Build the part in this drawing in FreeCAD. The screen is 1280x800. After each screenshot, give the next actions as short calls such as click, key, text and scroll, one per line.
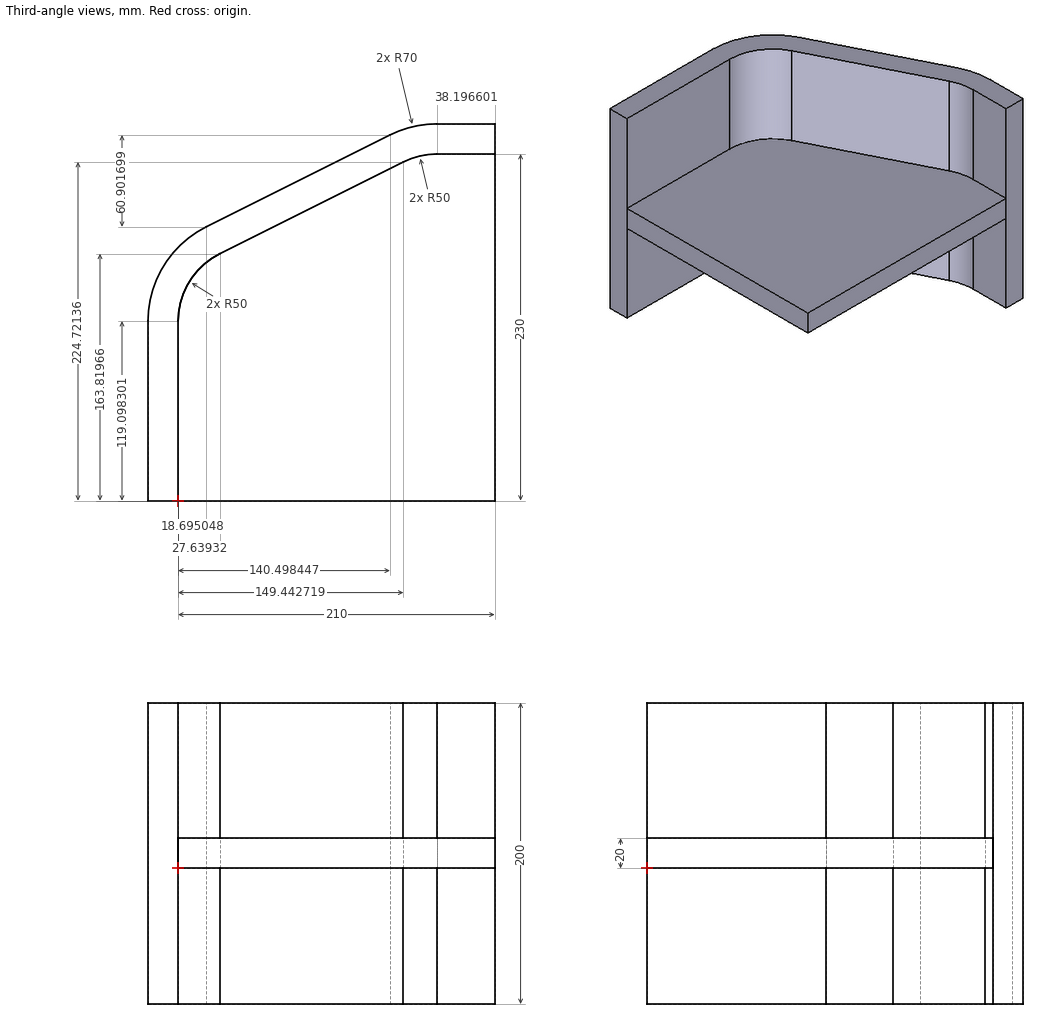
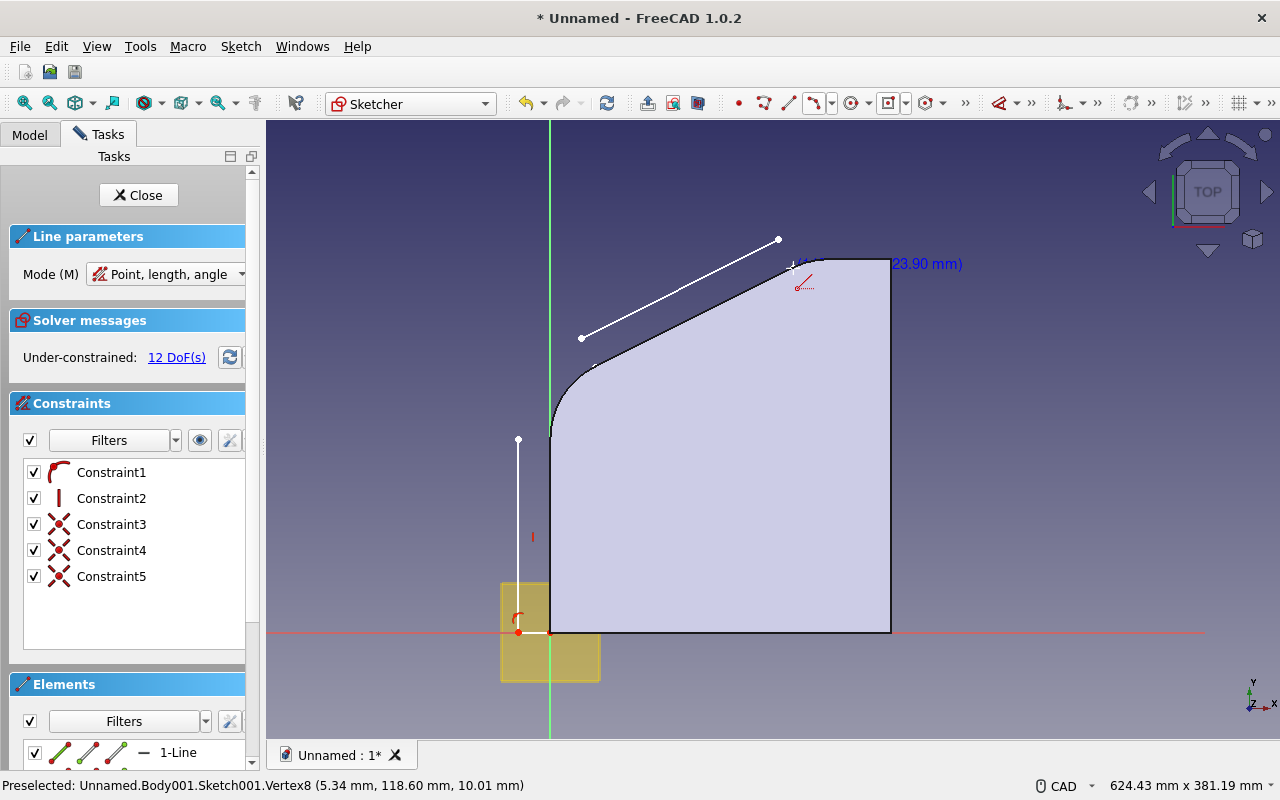
click(764, 104)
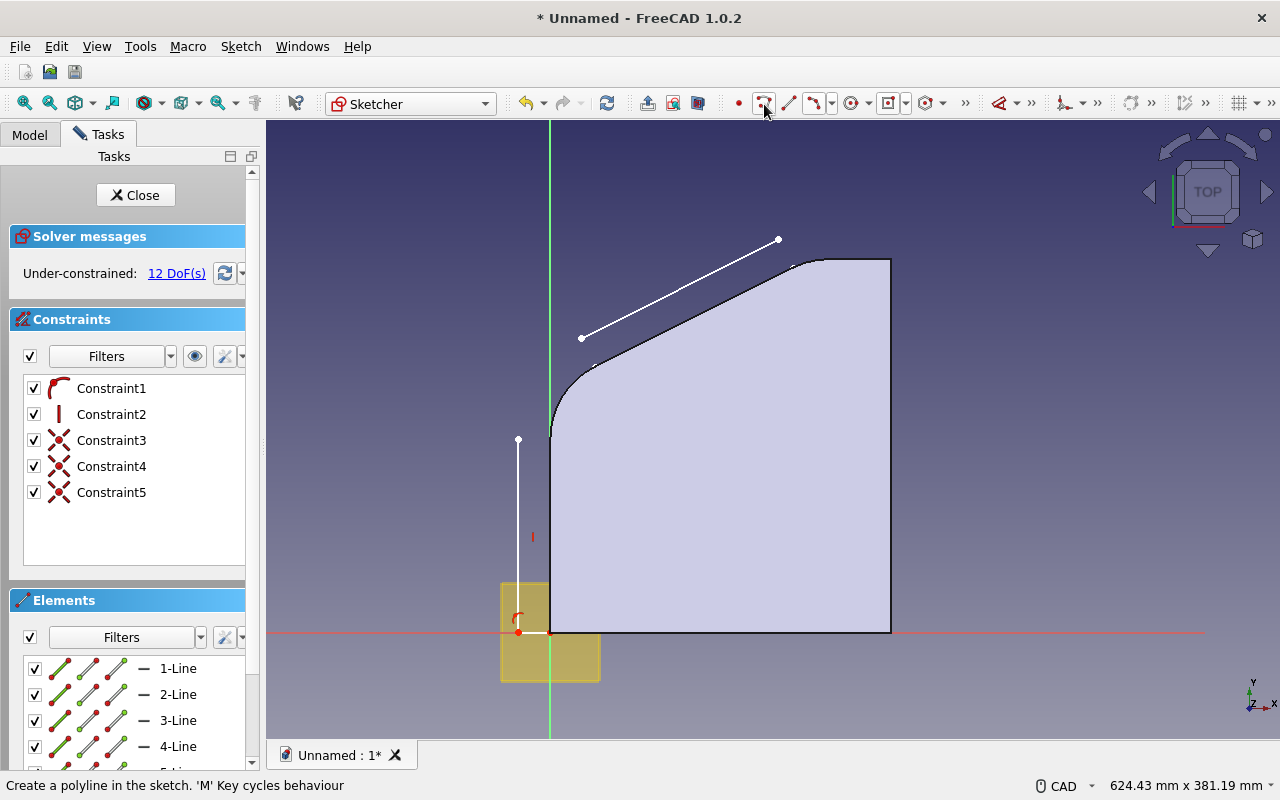
click(829, 259)
click(891, 259)
click(891, 227)
click(829, 227)
right_click(829, 227)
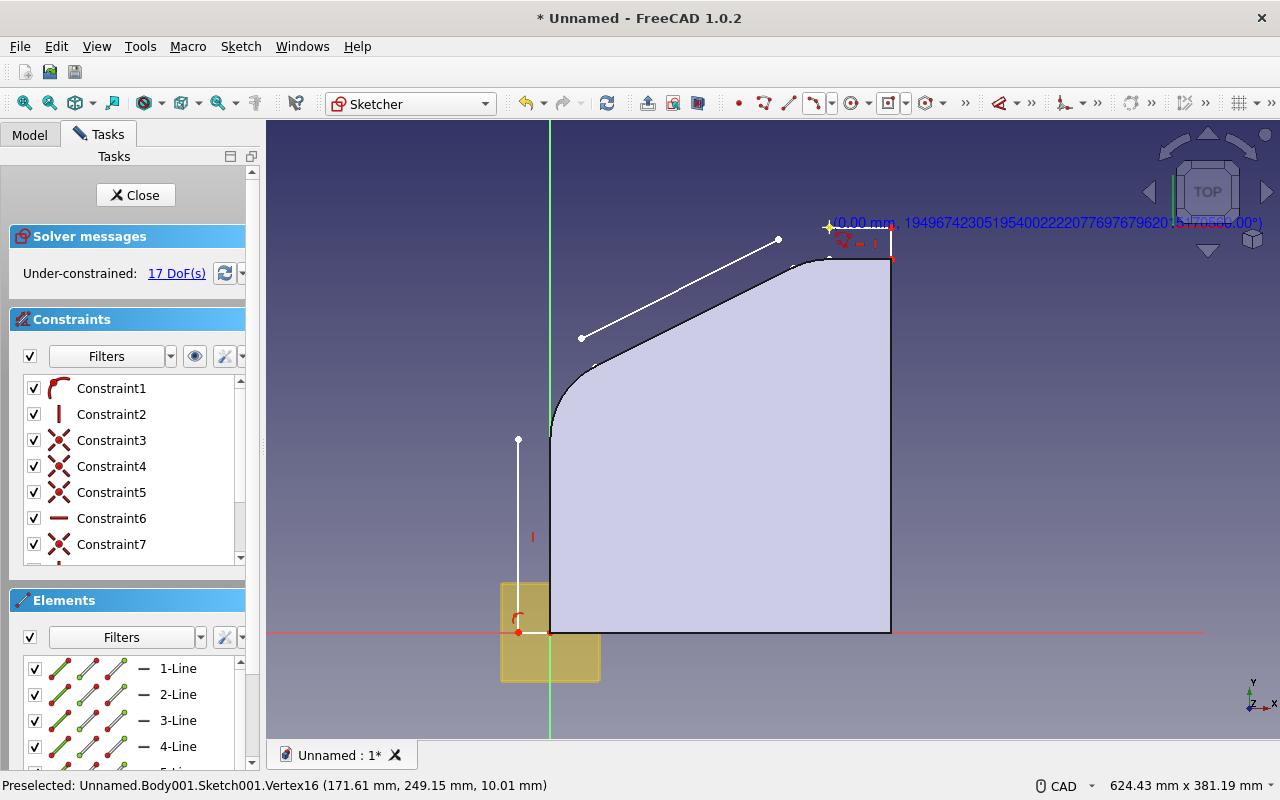
click(814, 104)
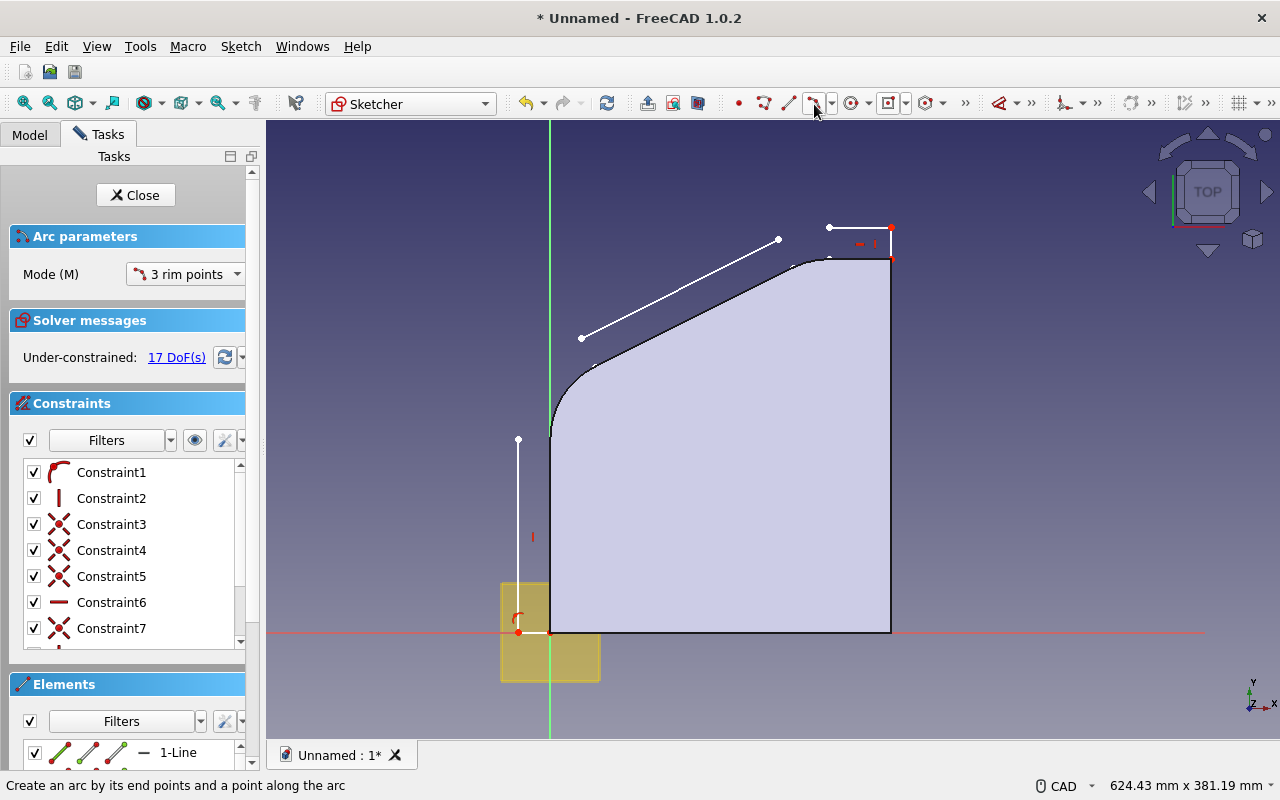
click(581, 339)
click(518, 440)
click(535, 379)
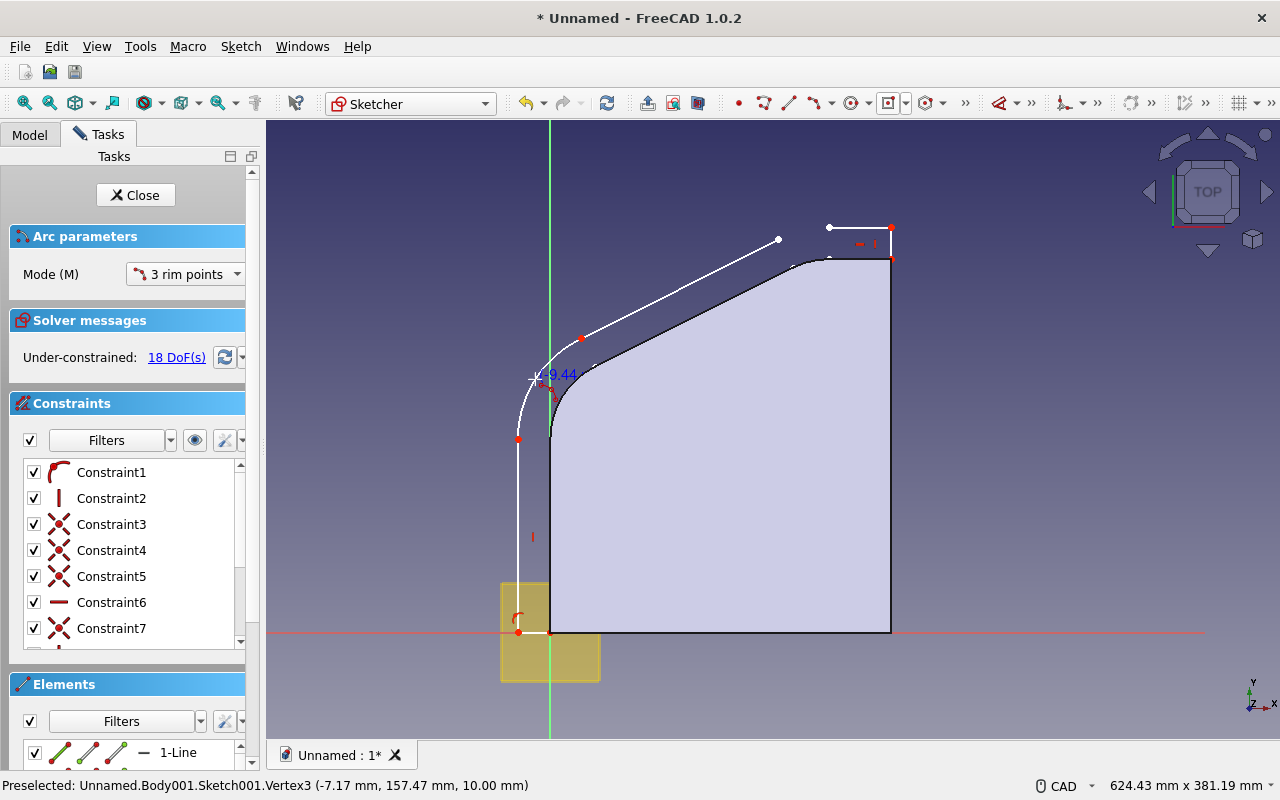
click(559, 440)
click(595, 368)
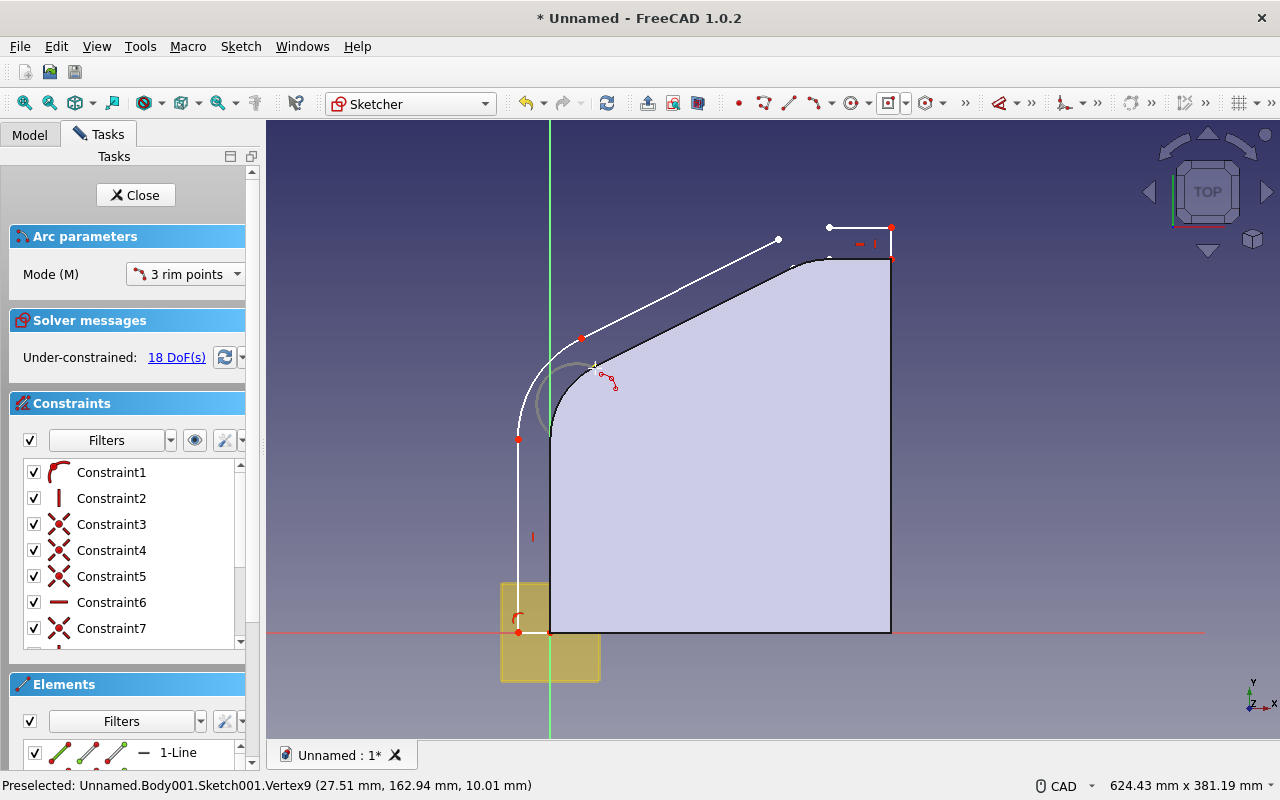
scroll(562, 396, up, 2)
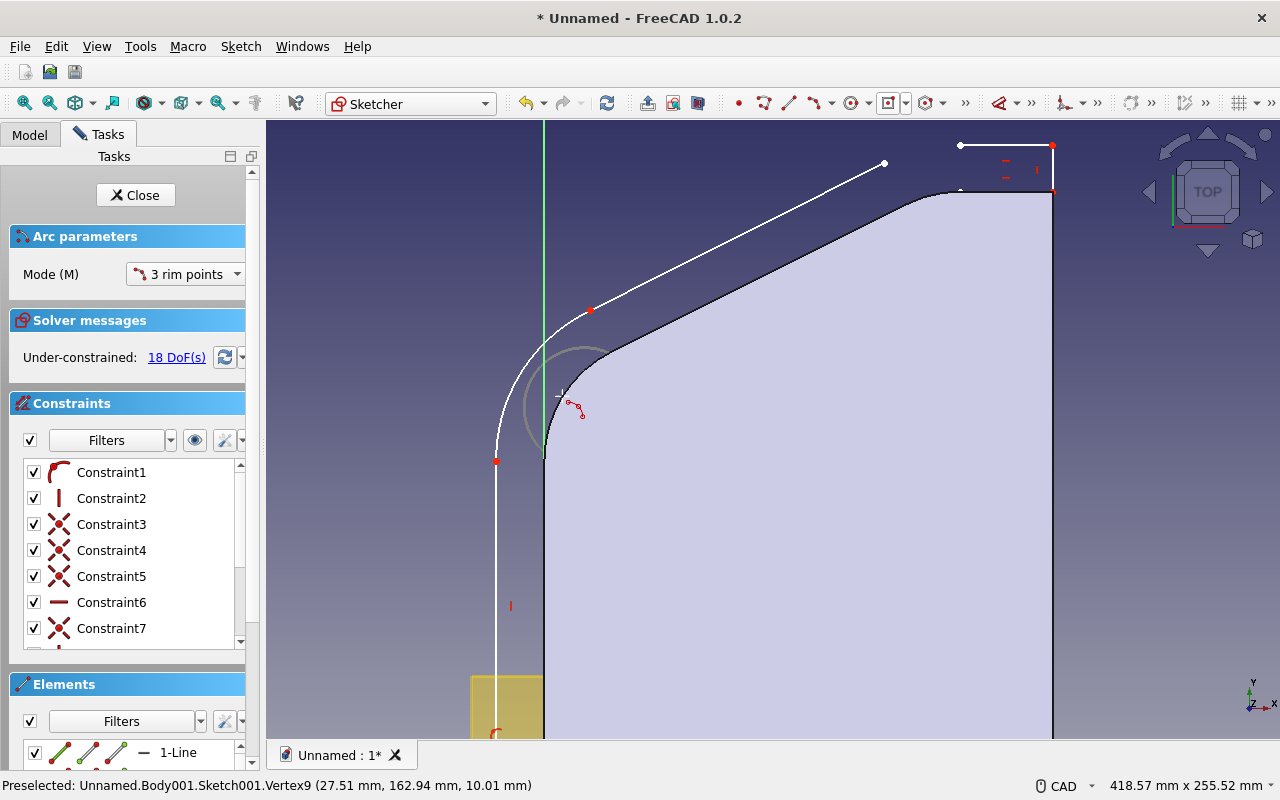
click(563, 397)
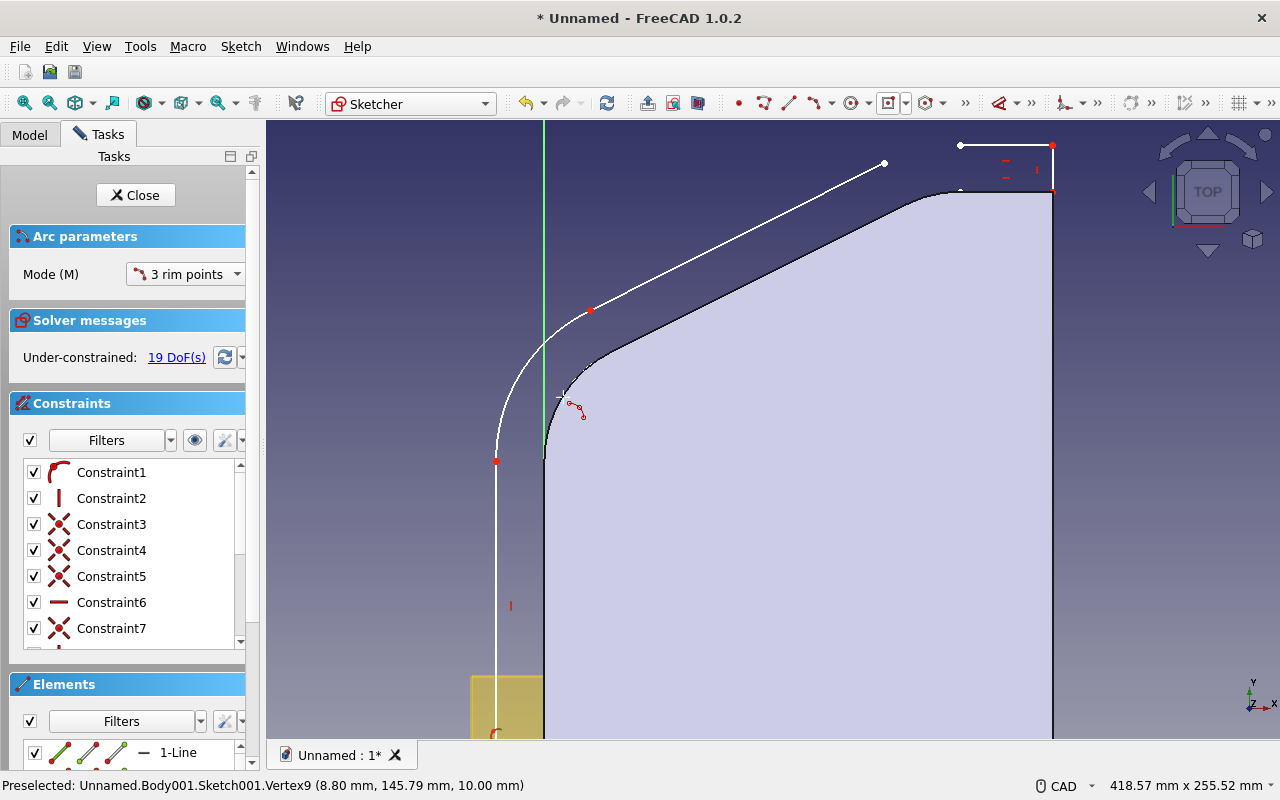
click(906, 206)
click(960, 193)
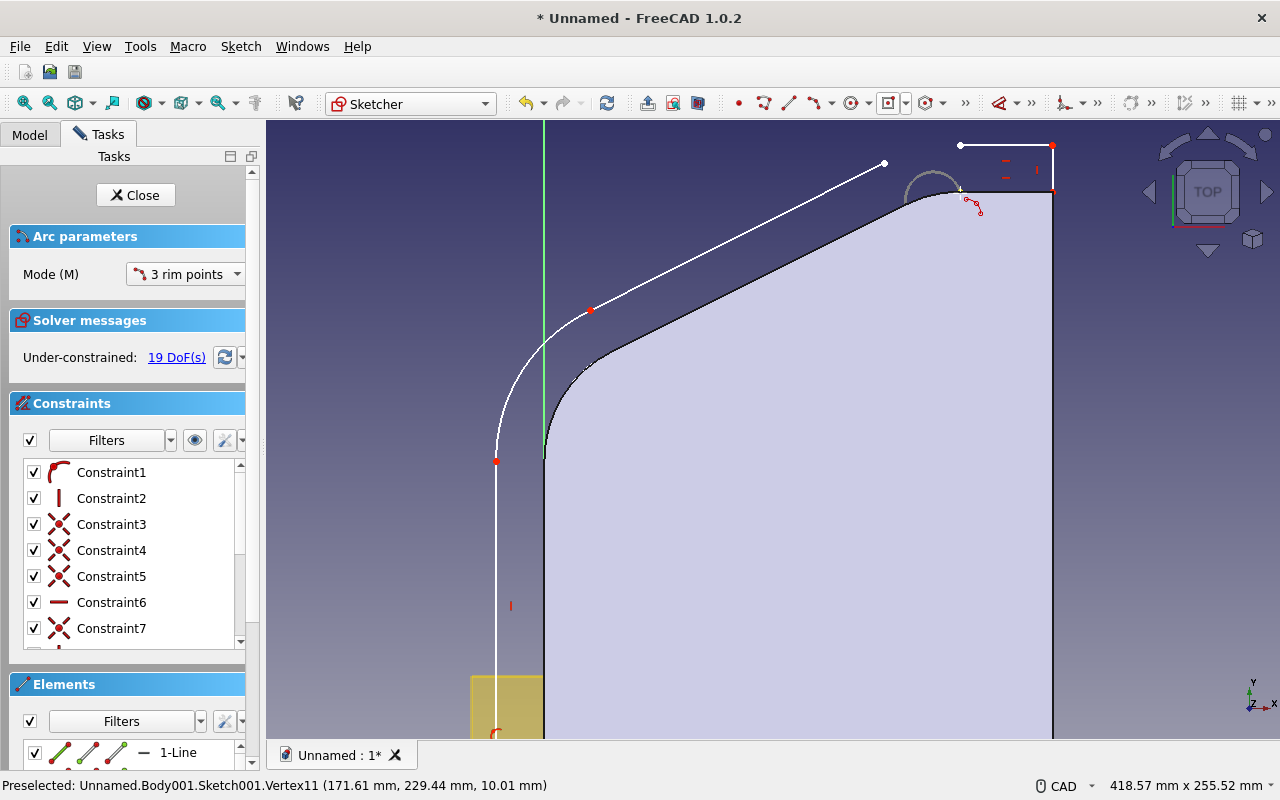
scroll(933, 195, up, 8)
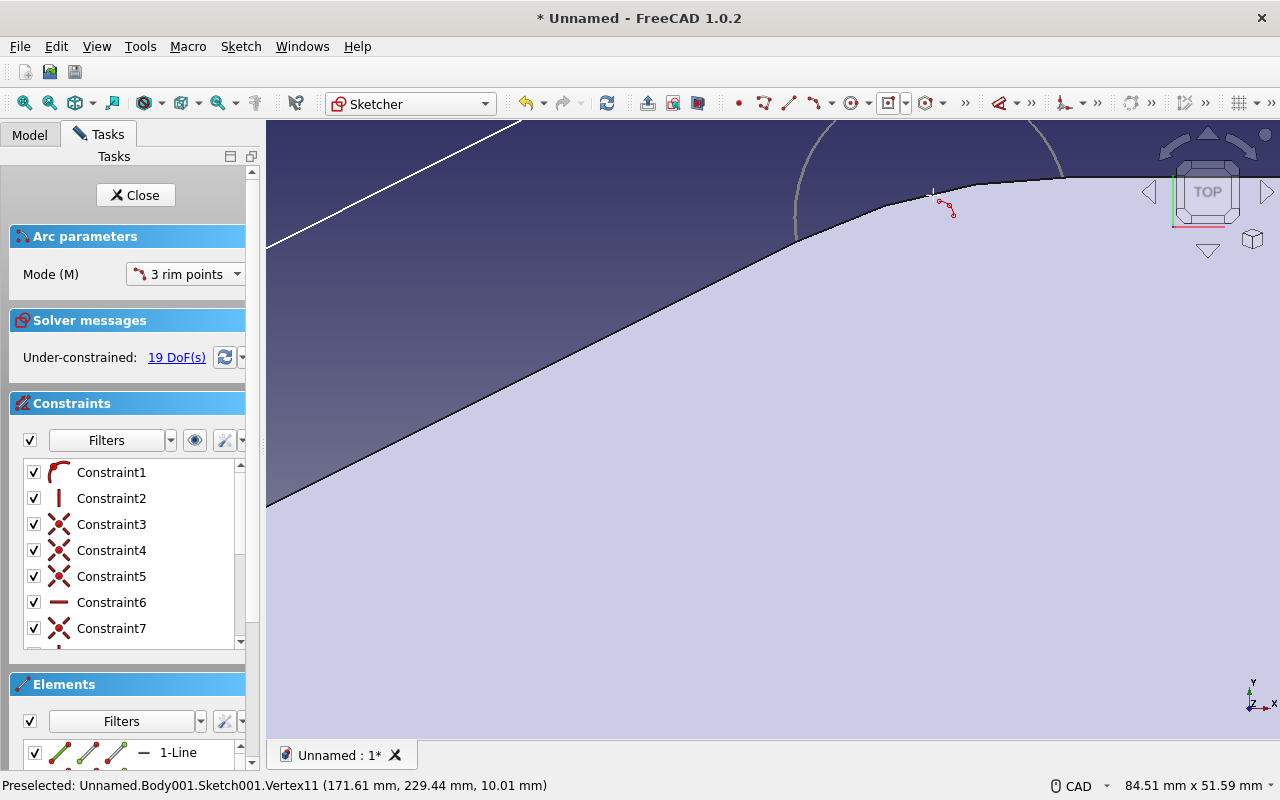
click(929, 193)